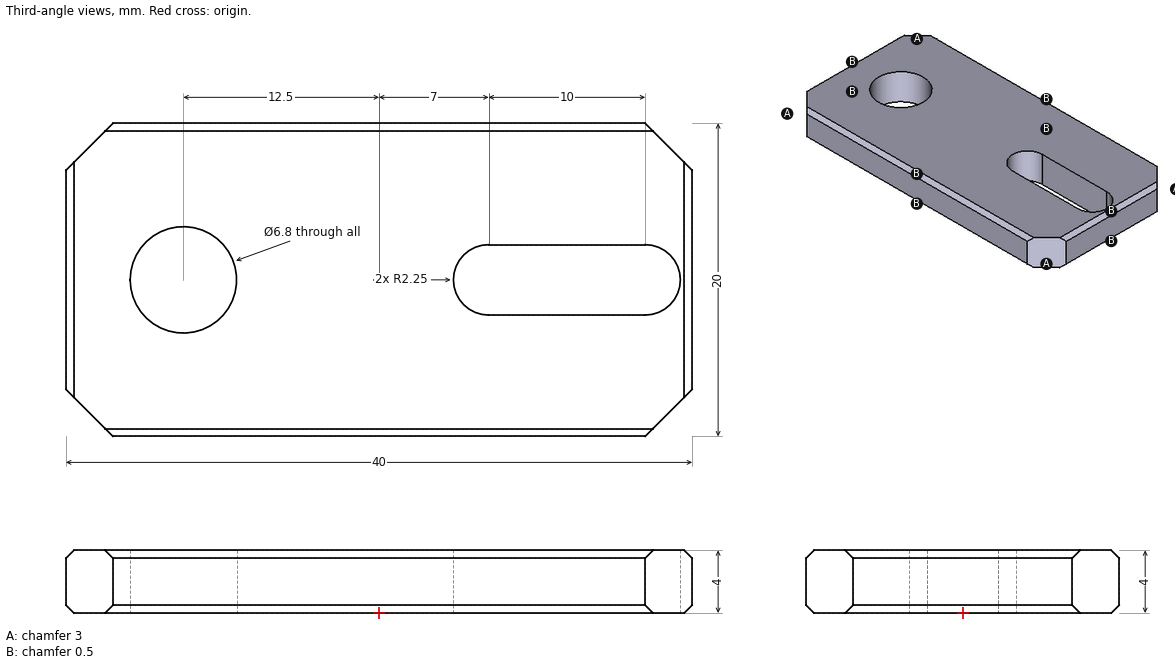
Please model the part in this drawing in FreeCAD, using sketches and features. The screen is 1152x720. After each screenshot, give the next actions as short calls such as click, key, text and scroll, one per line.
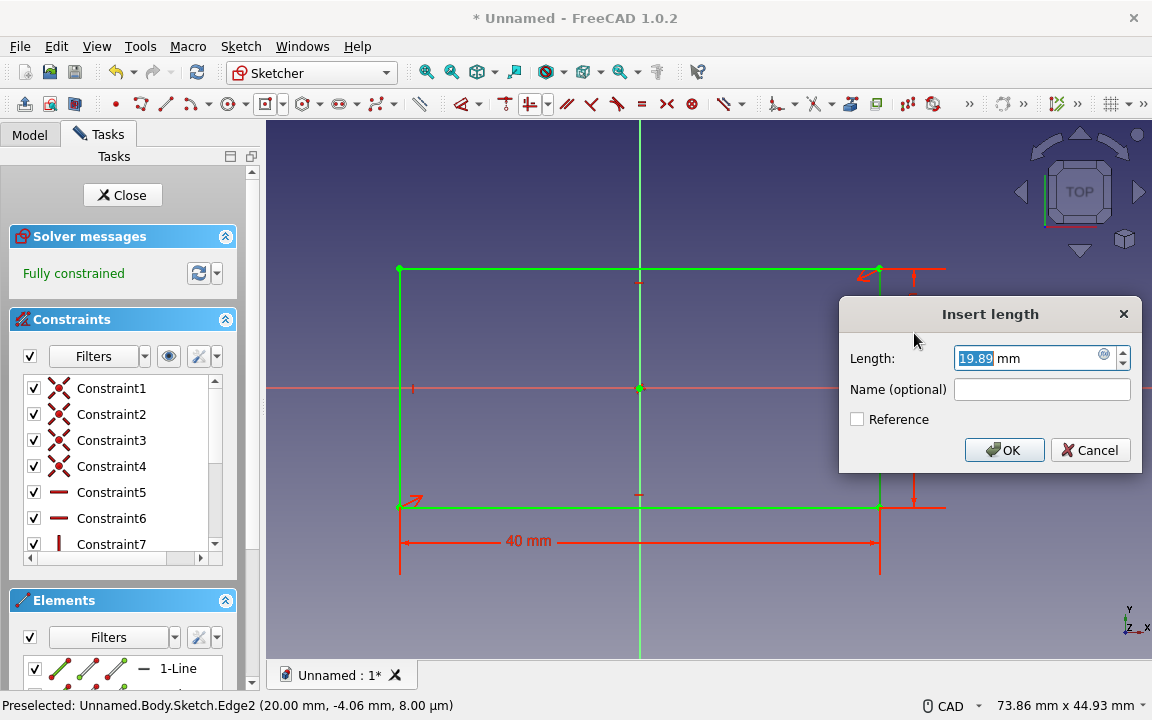
text(20)
key(Return)
key(Escape)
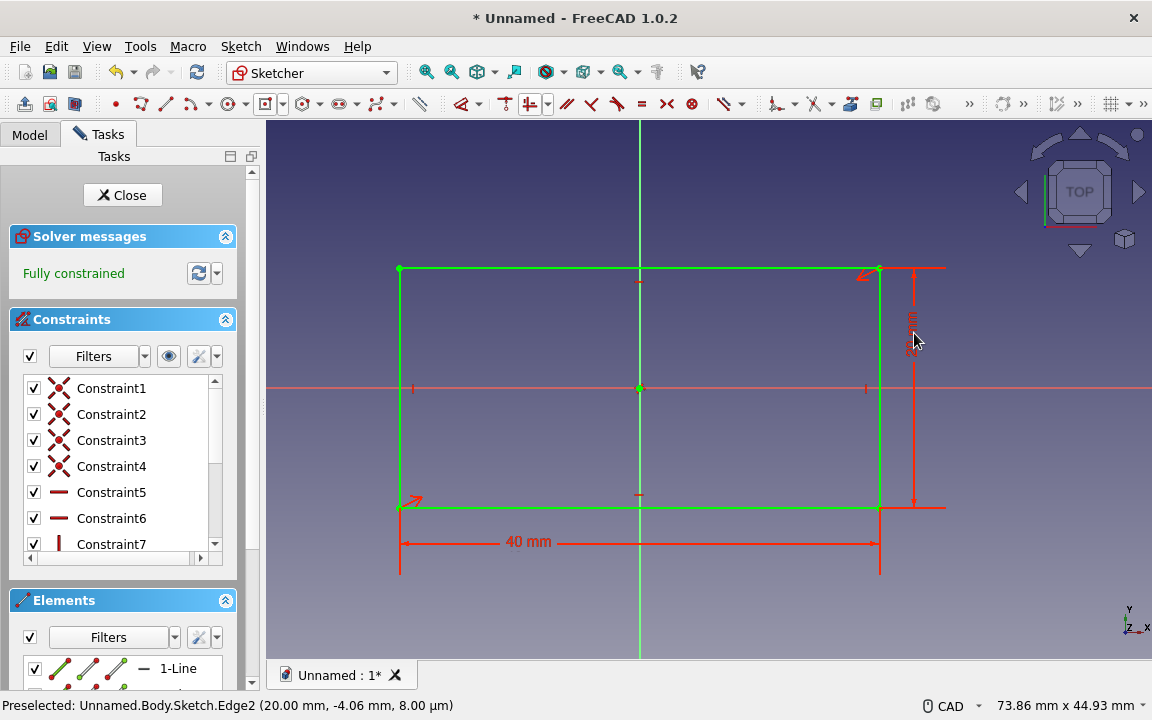
click(123, 195)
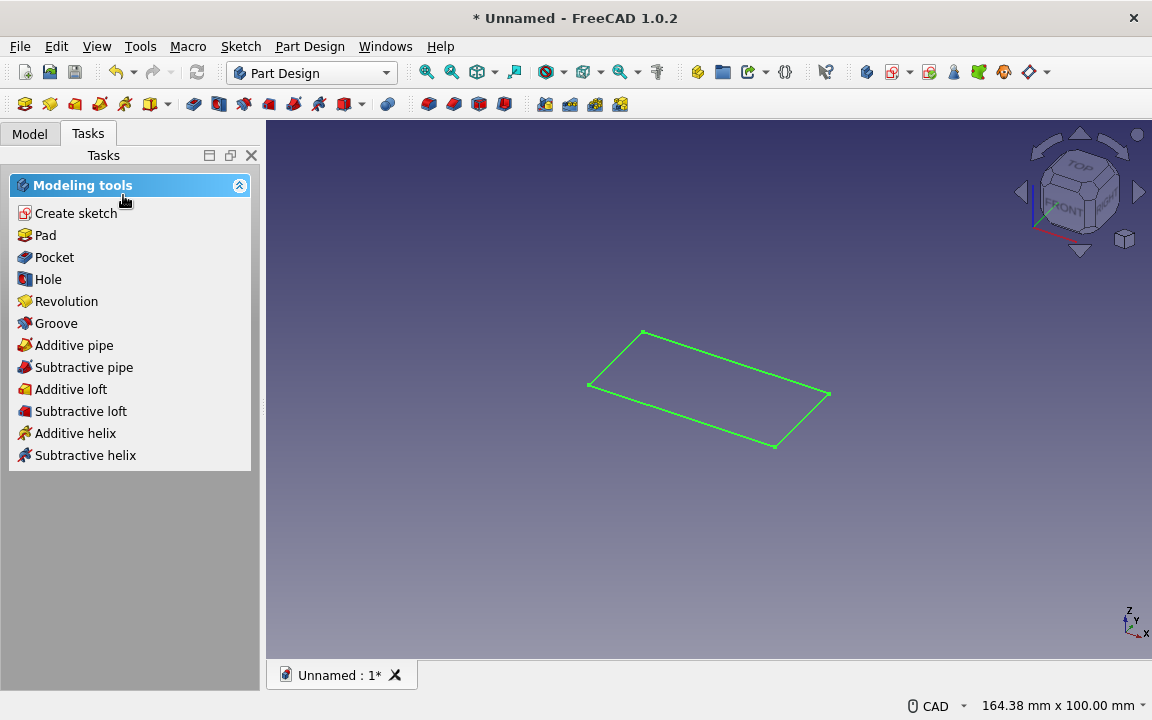
click(25, 104)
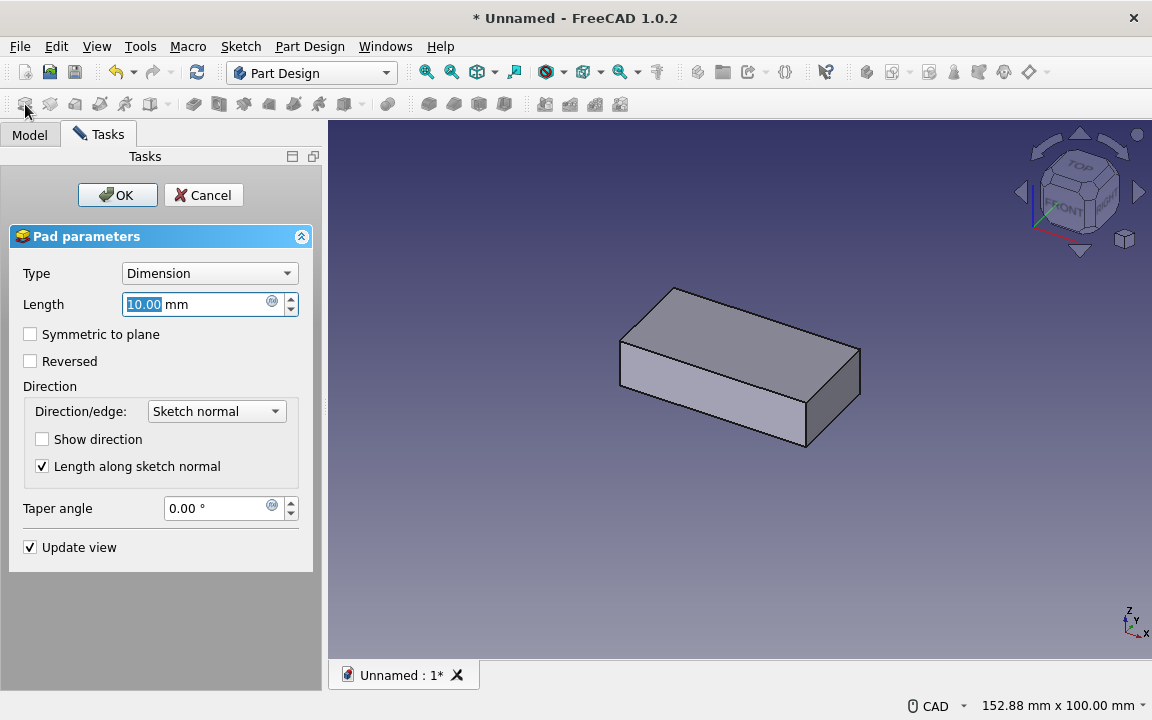
text(4)
key(Tab)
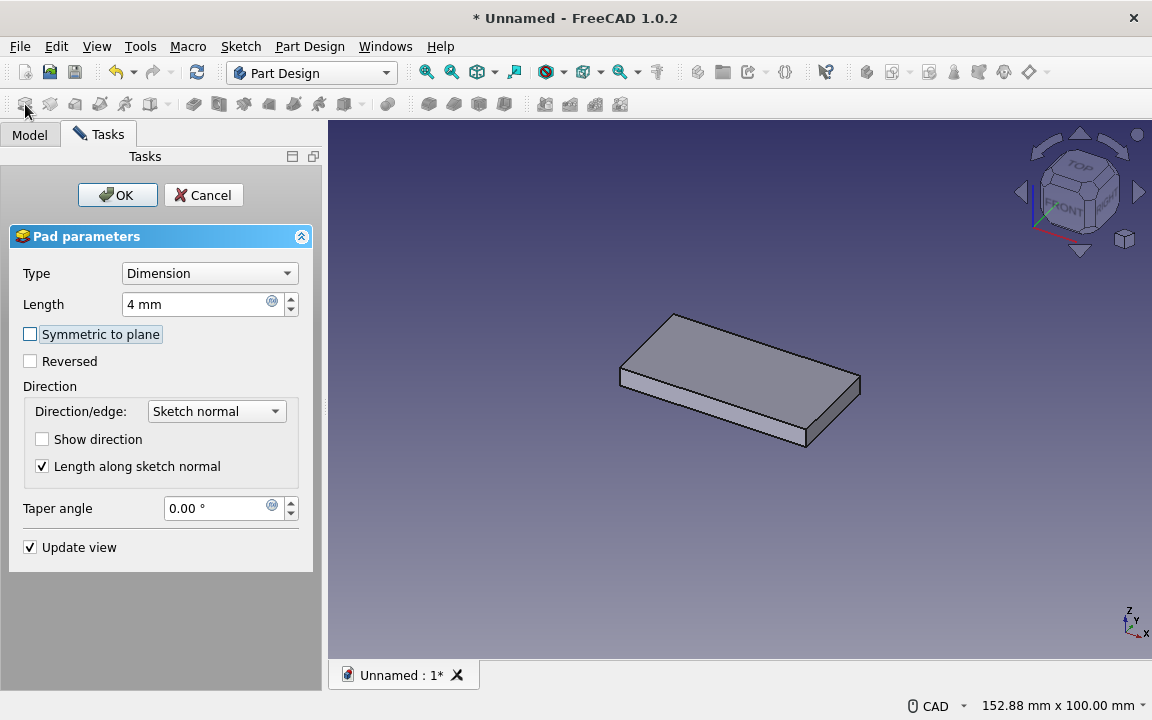
click(118, 195)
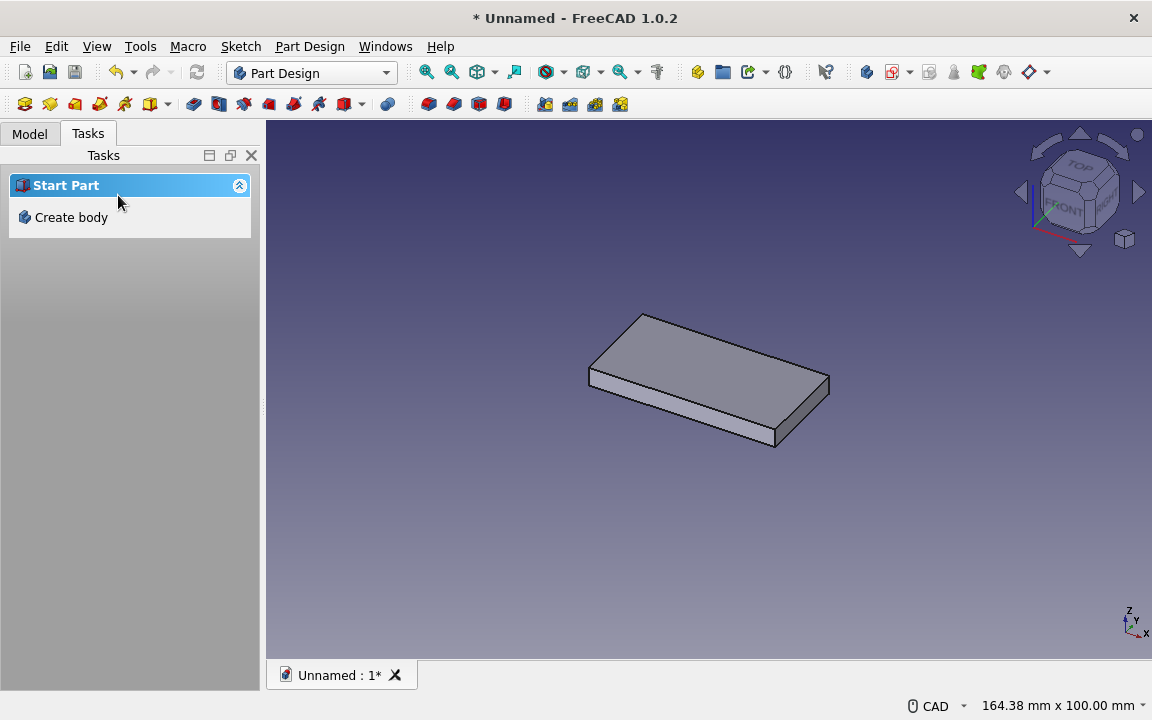
click(427, 72)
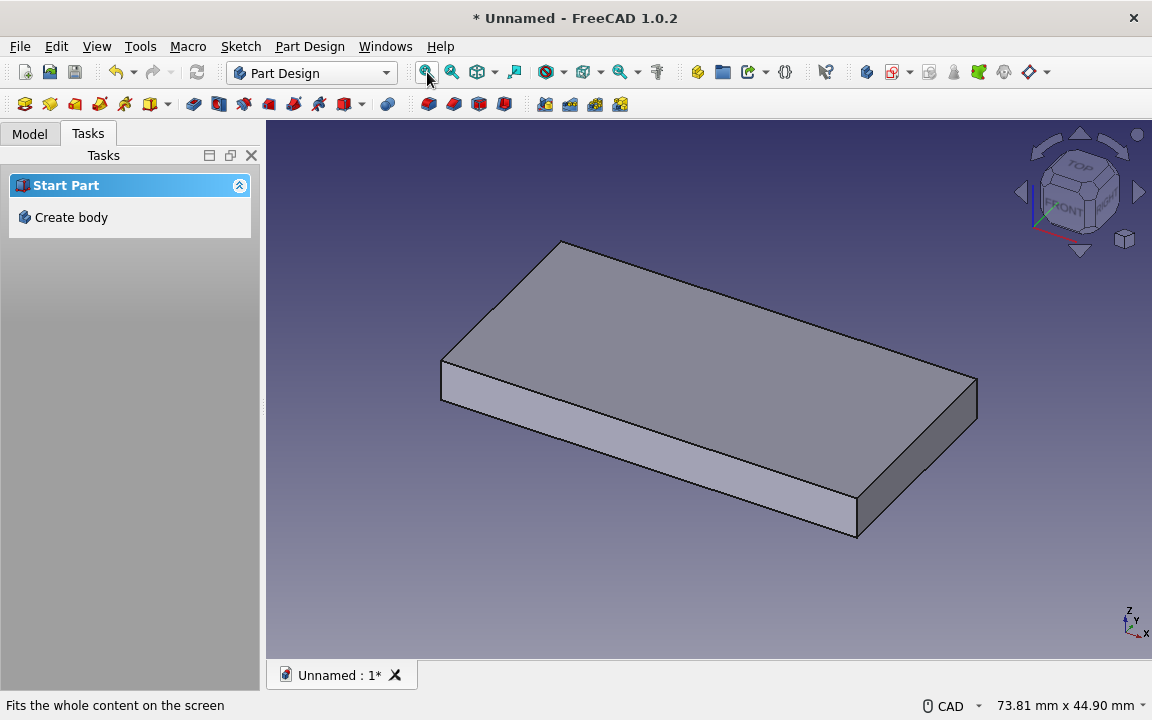
click(768, 389)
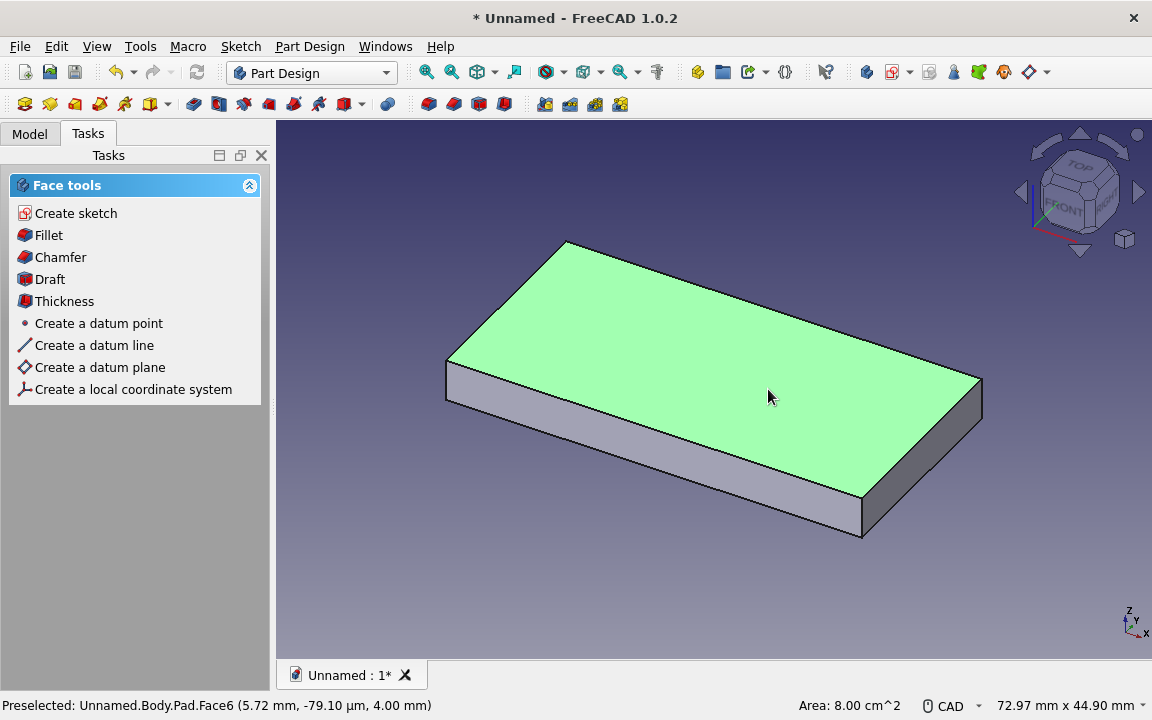
click(892, 72)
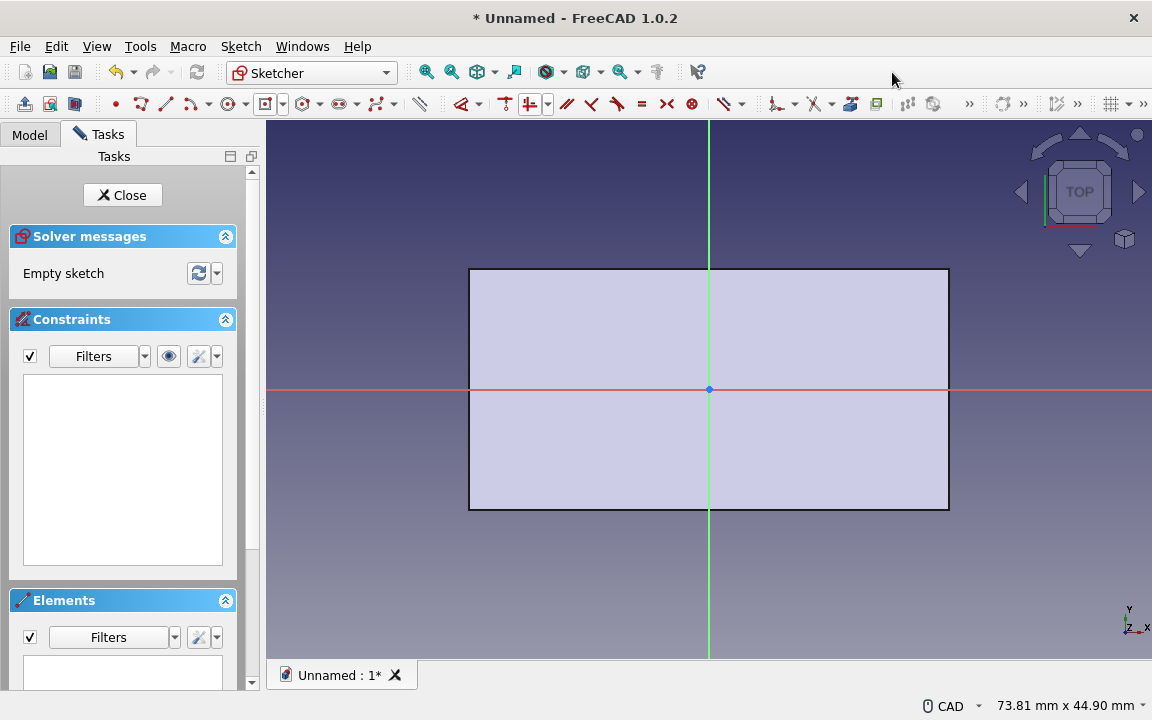
scroll(598, 390, up, 5)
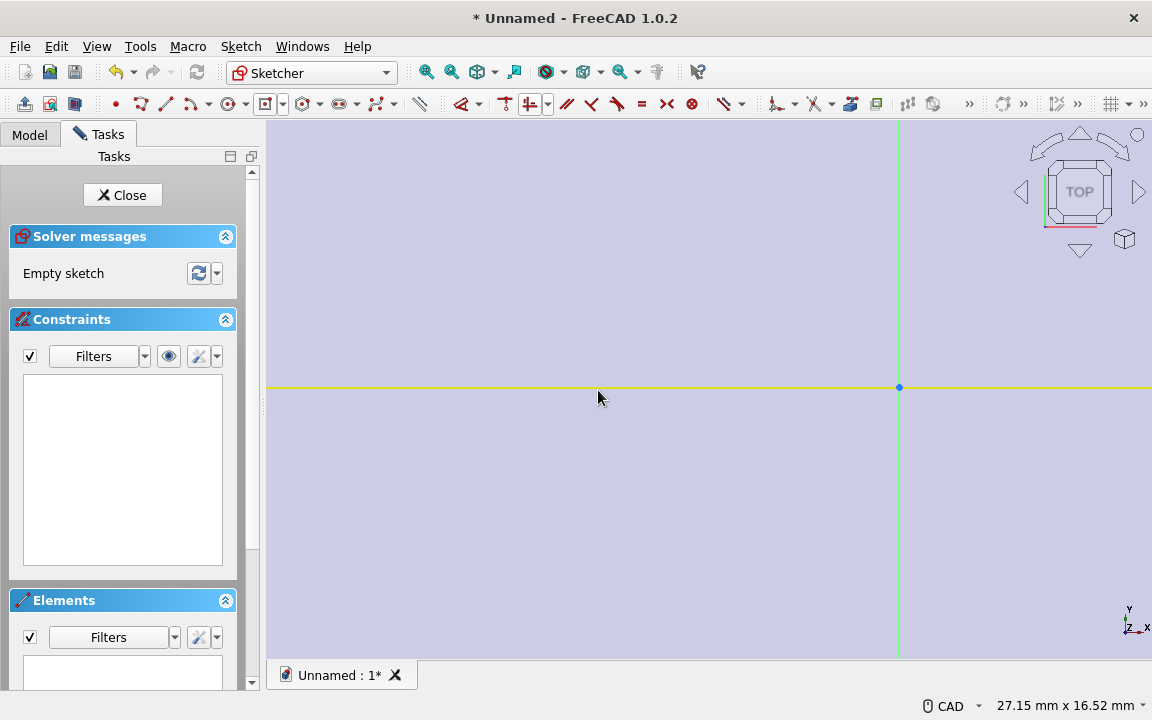
click(228, 104)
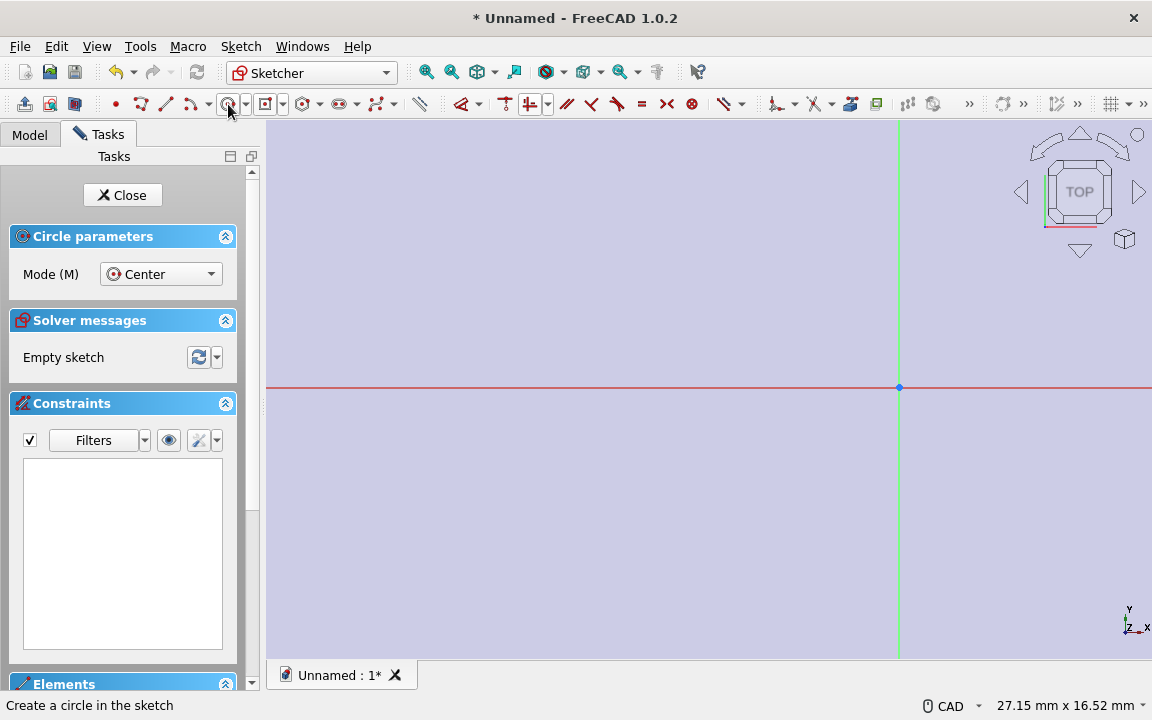
click(491, 388)
click(570, 309)
key(Escape)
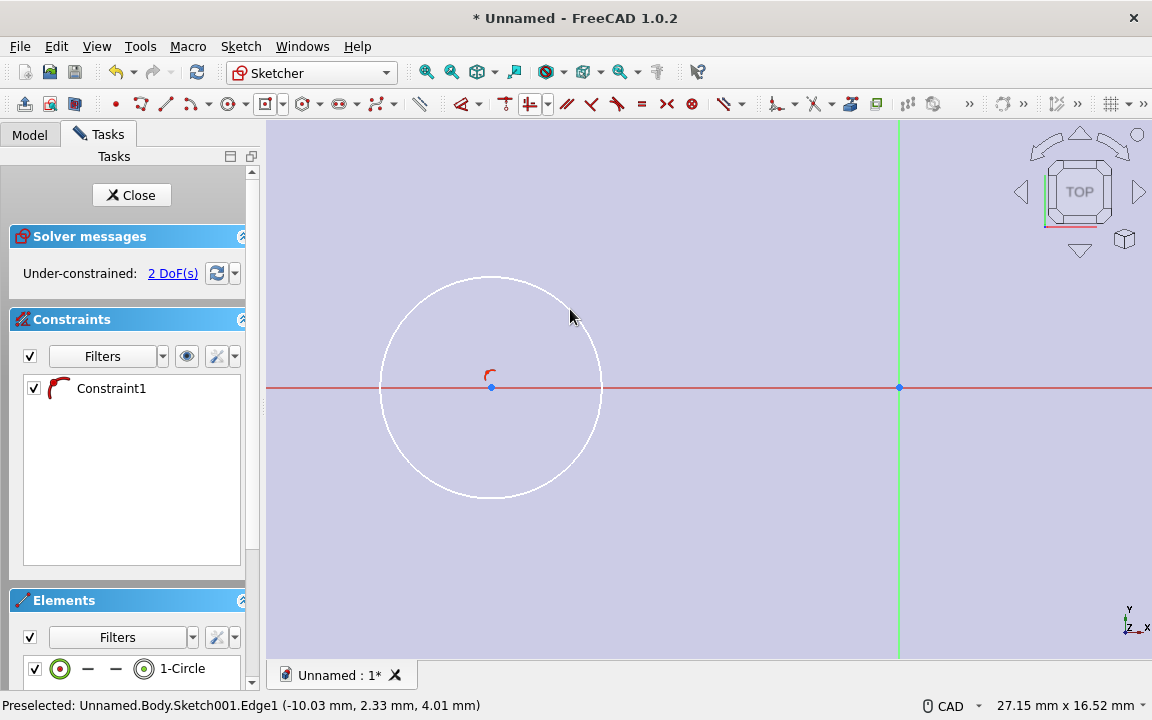
click(460, 104)